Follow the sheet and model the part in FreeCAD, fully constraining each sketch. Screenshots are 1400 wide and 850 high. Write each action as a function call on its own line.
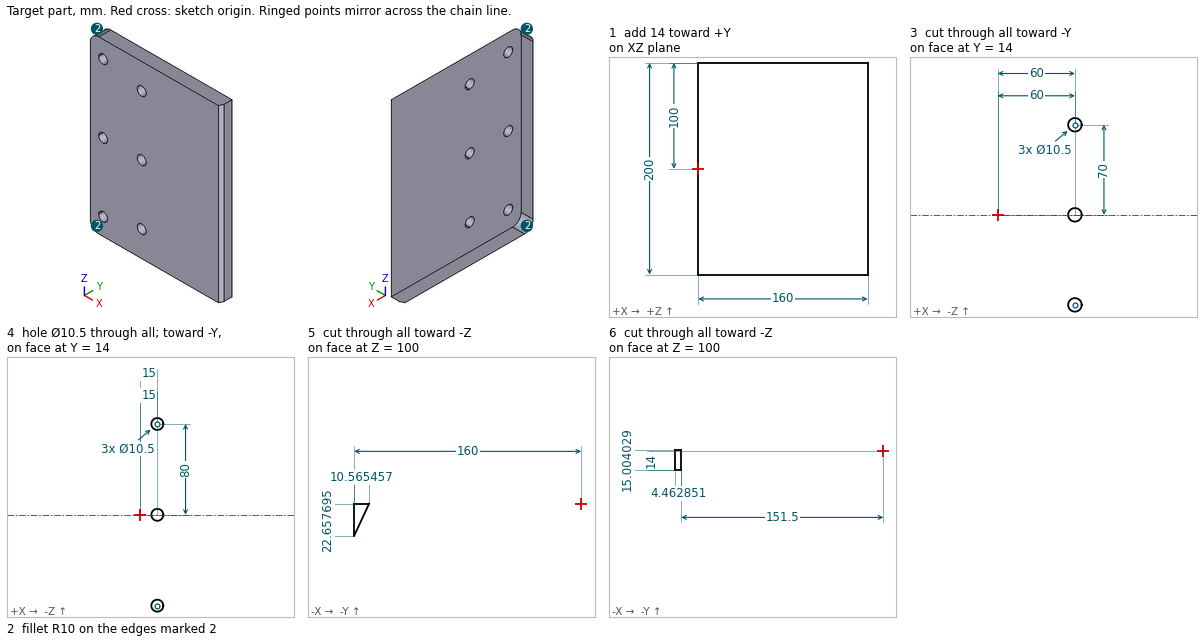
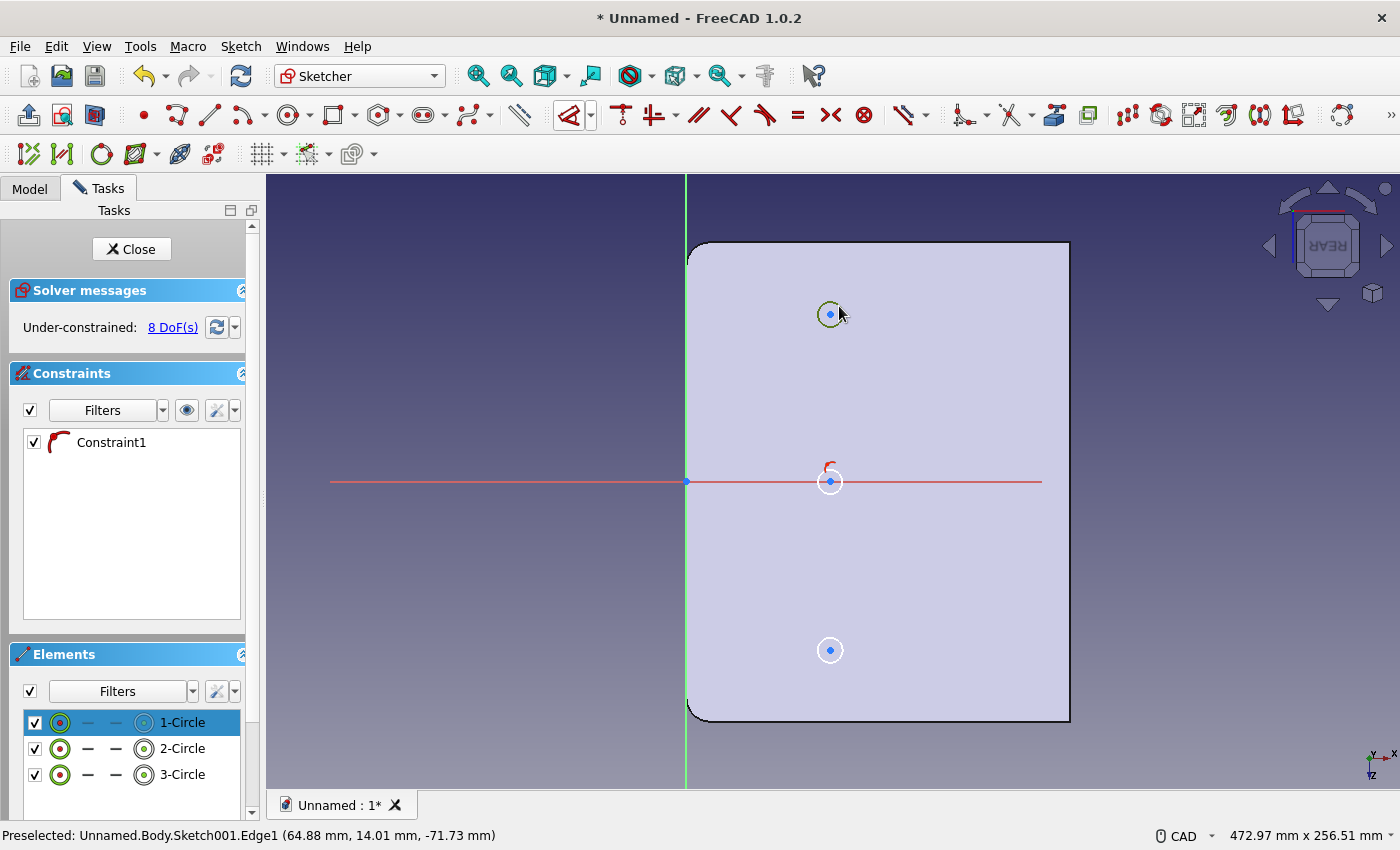
click(839, 642)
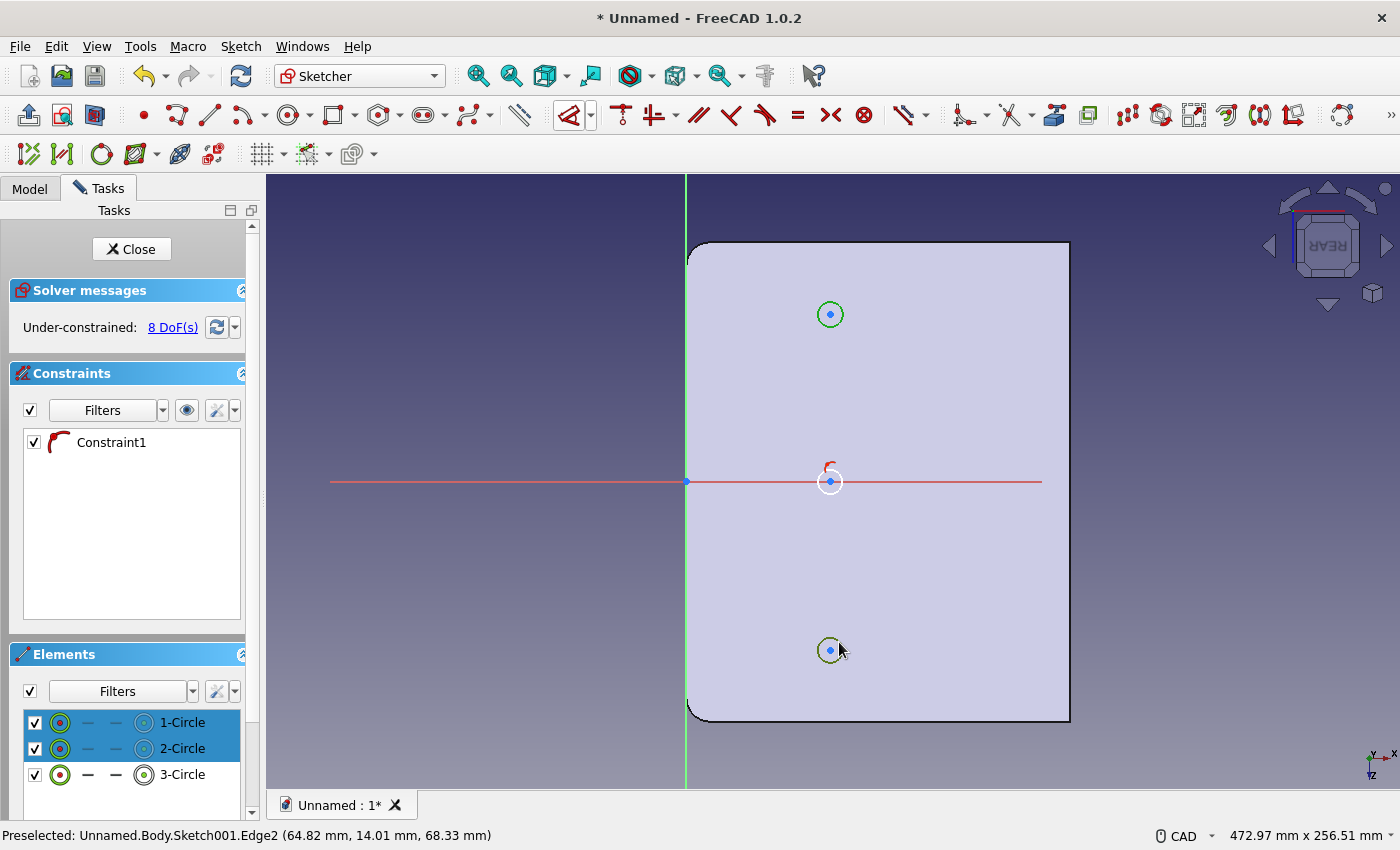
click(818, 482)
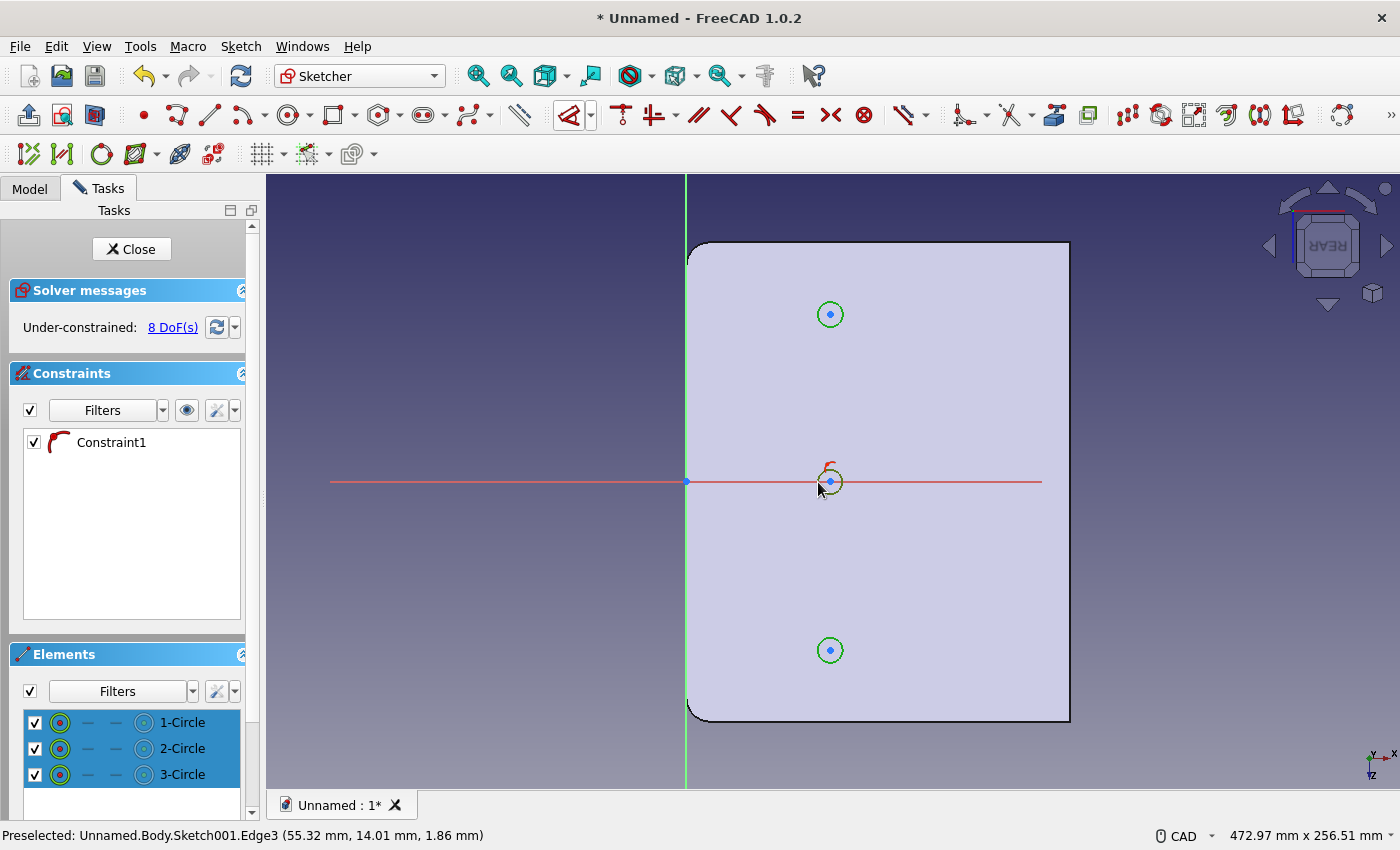
click(798, 116)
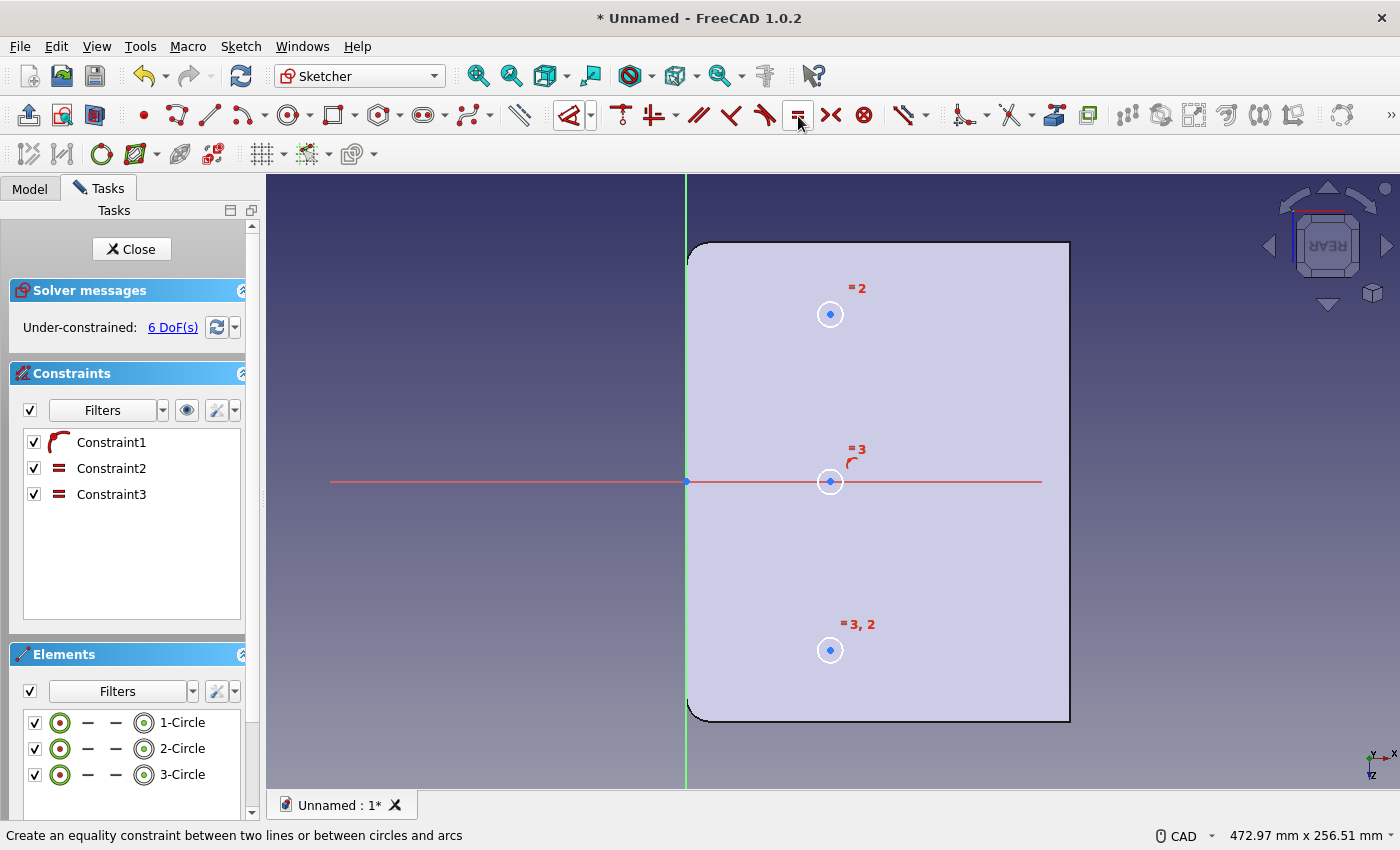
click(830, 315)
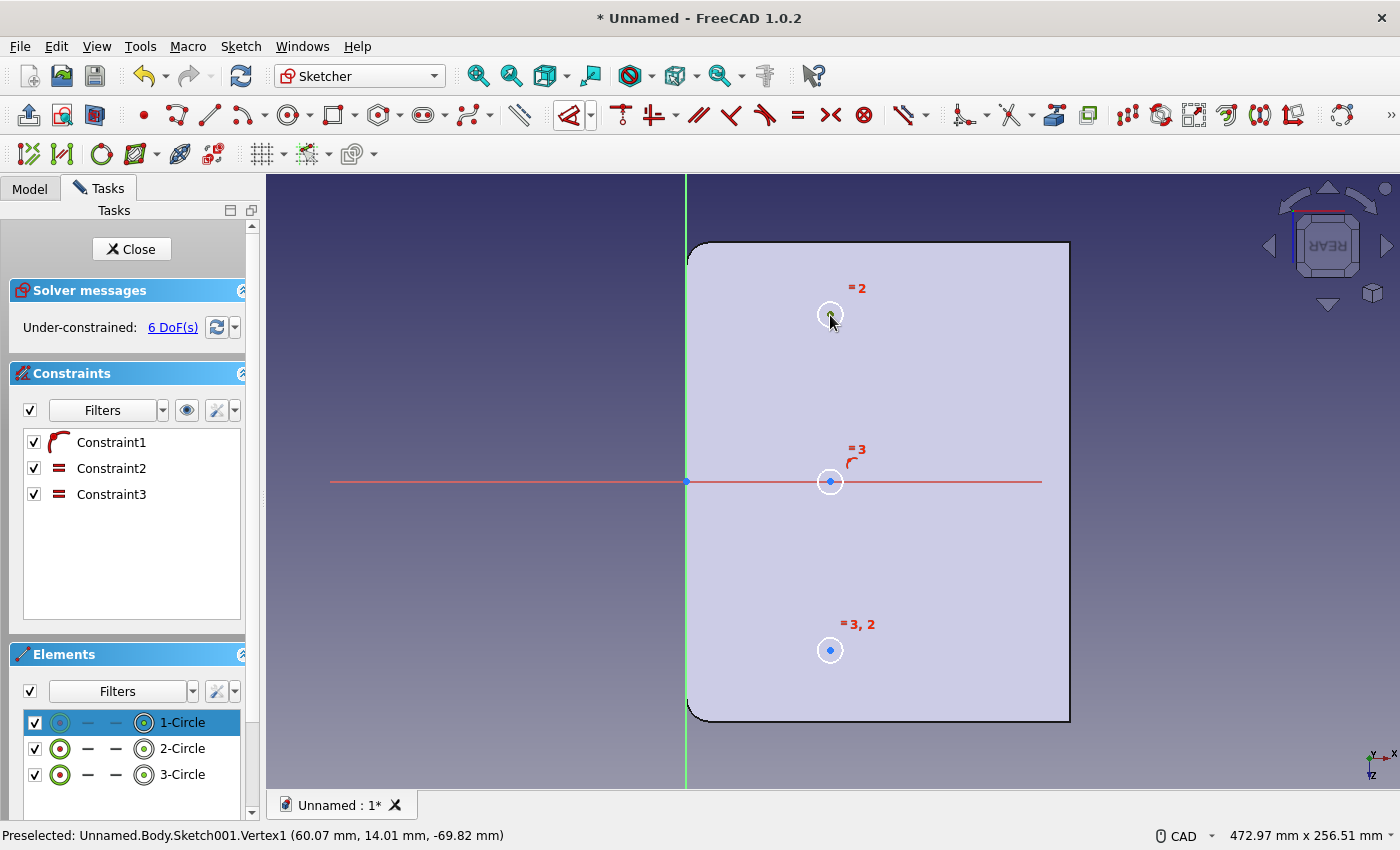
click(830, 650)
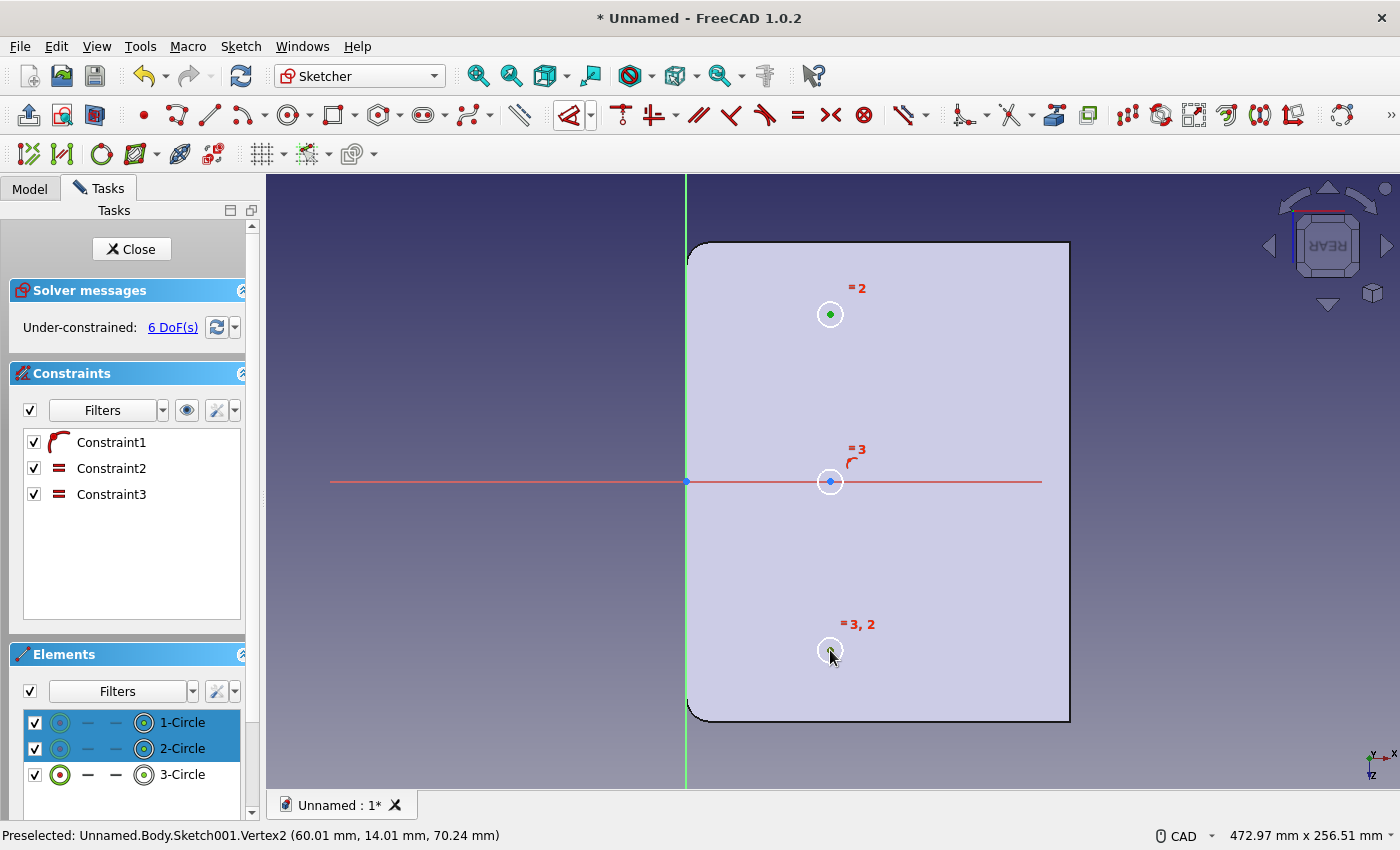
click(361, 482)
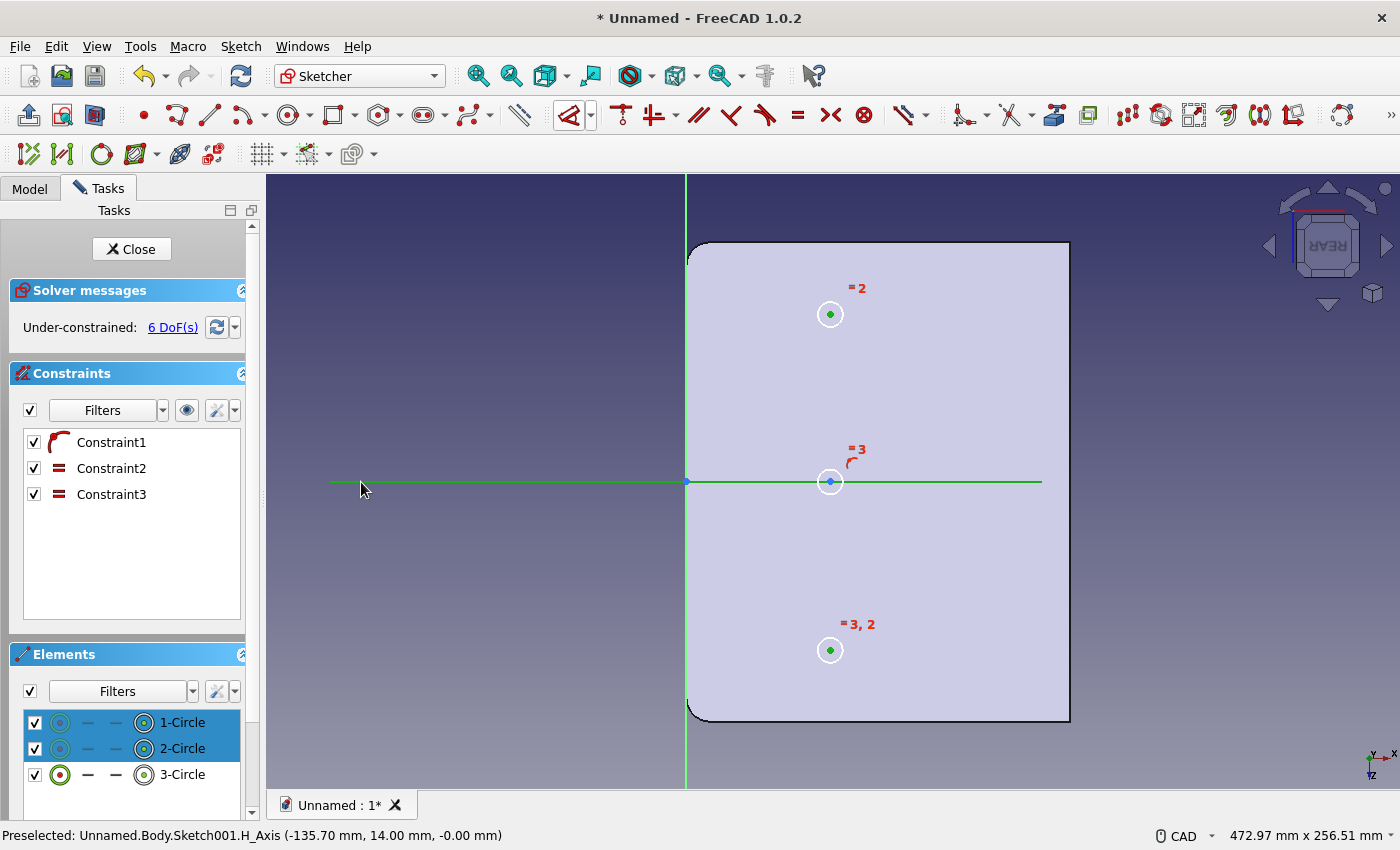
click(831, 116)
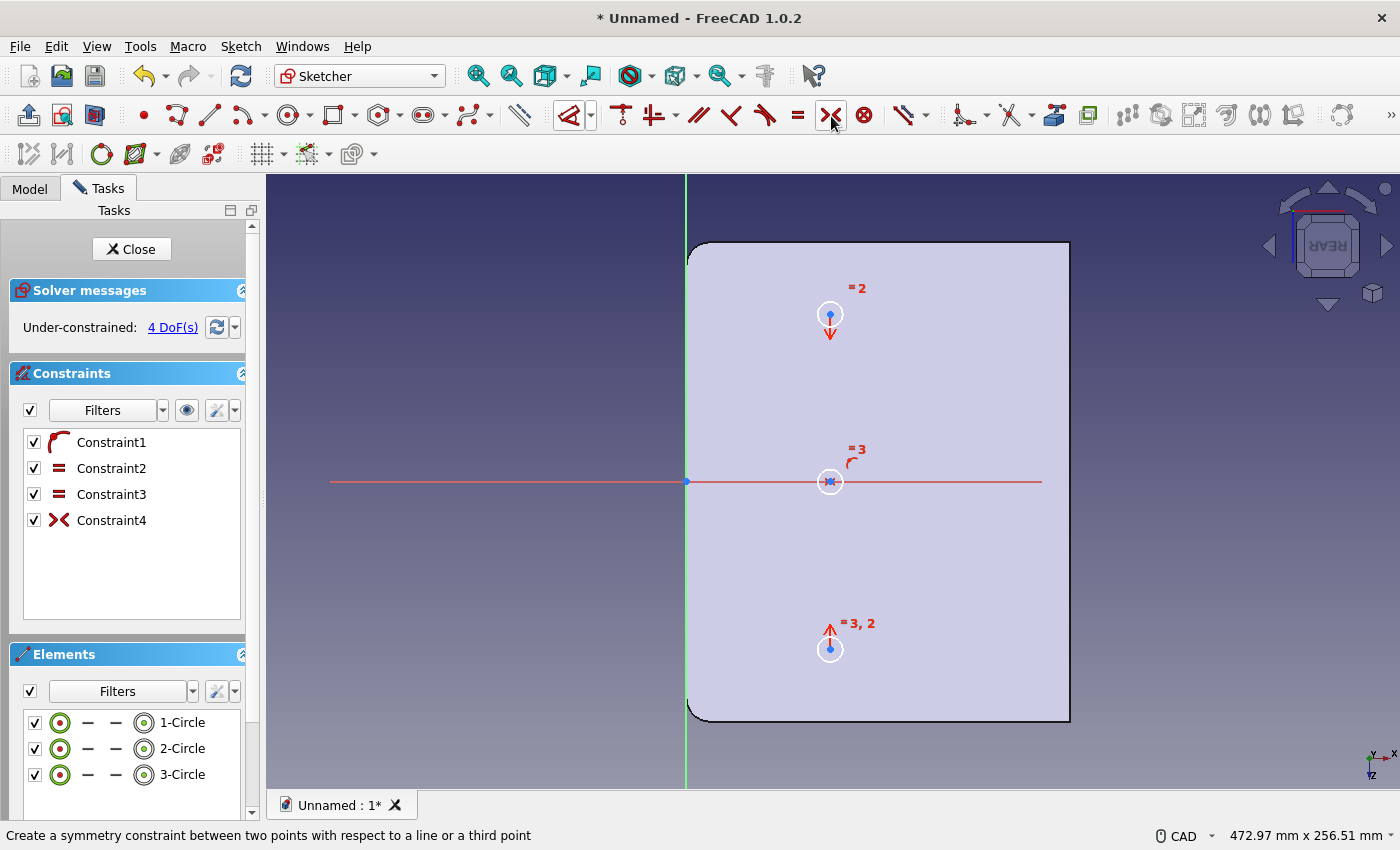
click(568, 116)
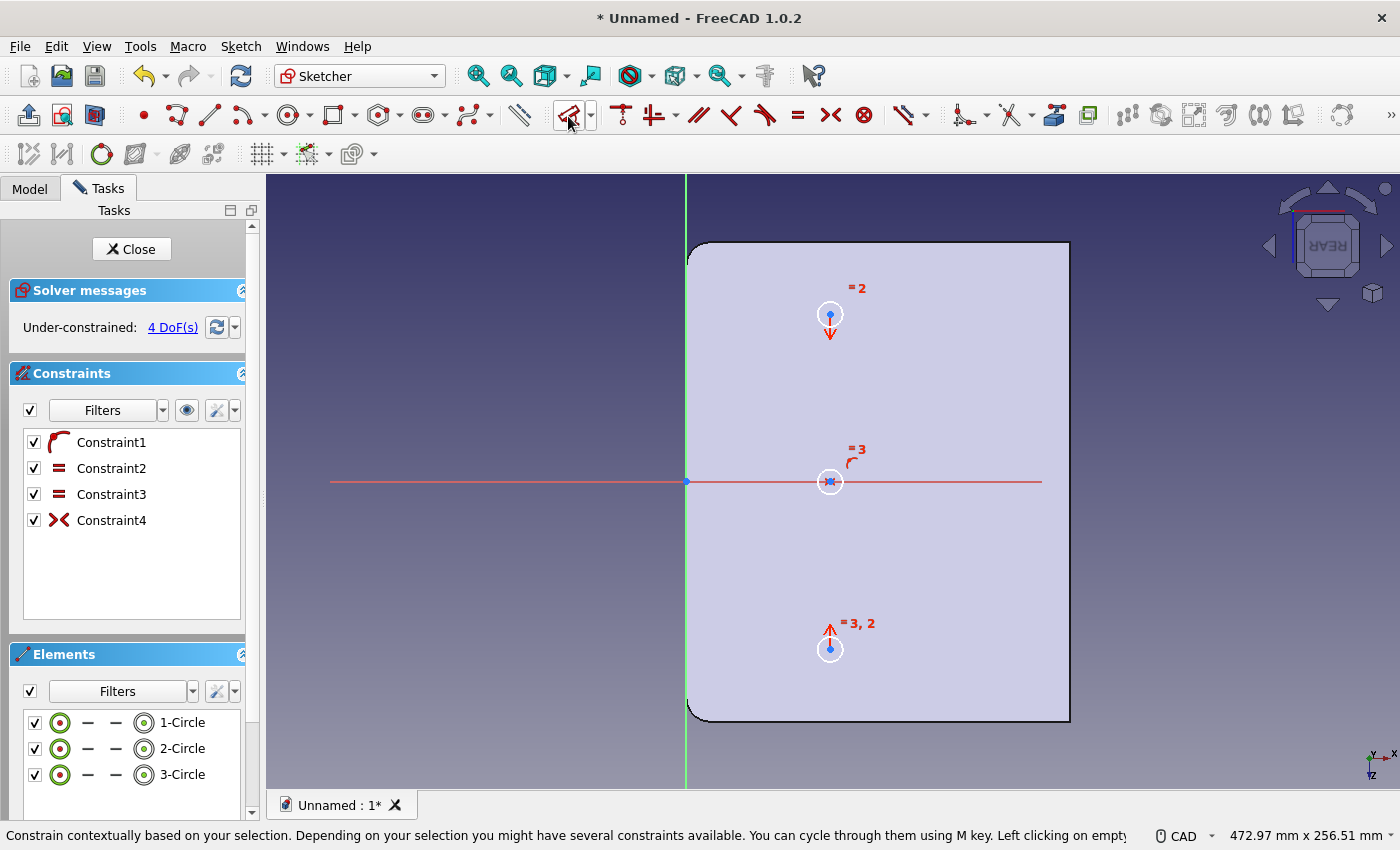
scroll(839, 306, up, 3)